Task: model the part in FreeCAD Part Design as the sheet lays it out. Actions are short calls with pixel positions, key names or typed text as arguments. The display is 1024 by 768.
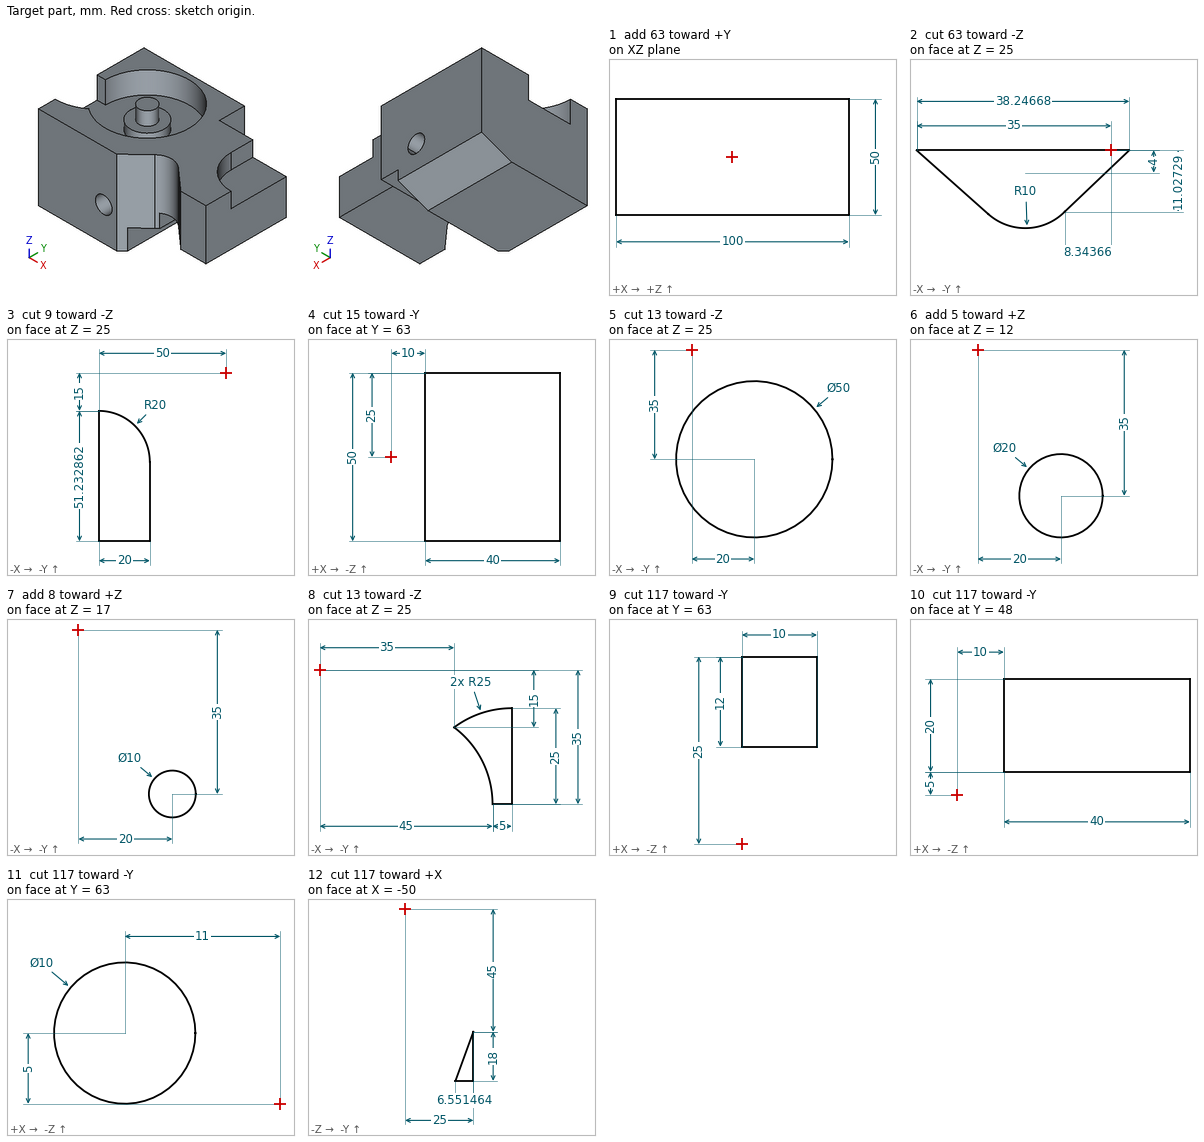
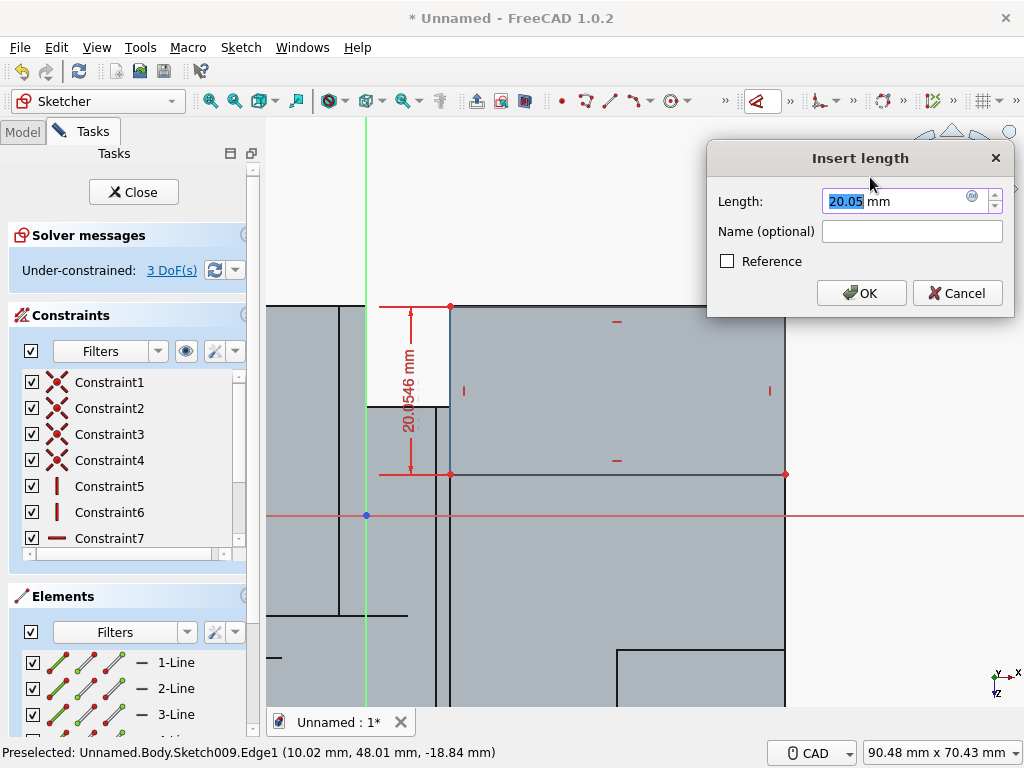
text(20)
key(Return)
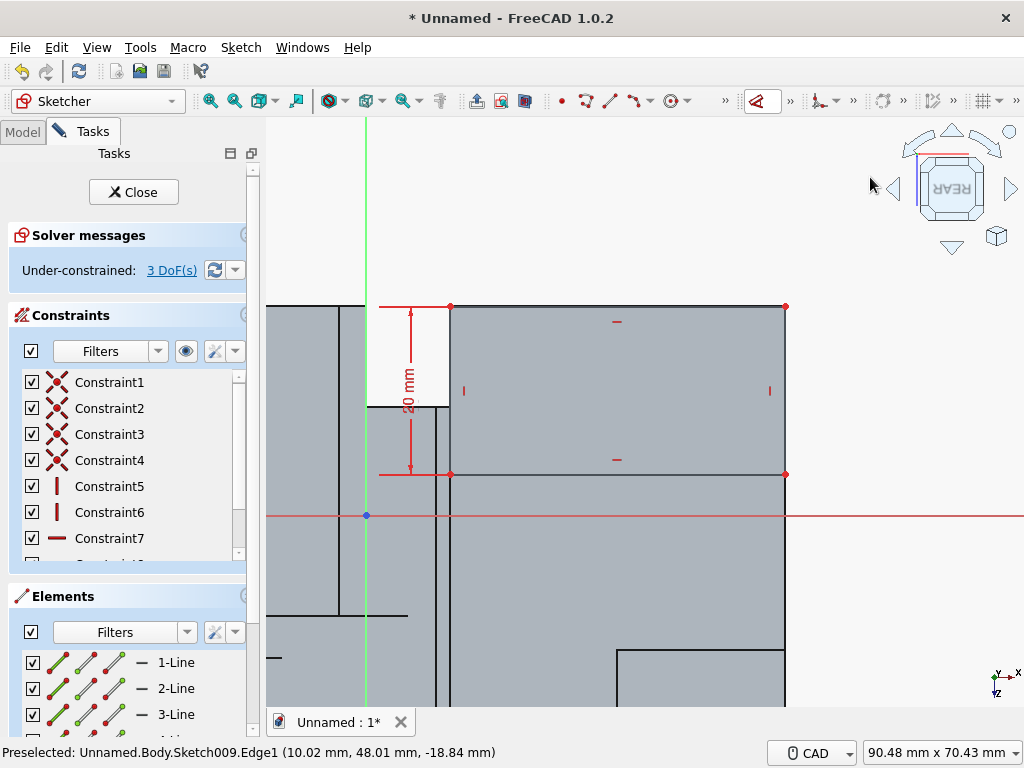
click(550, 475)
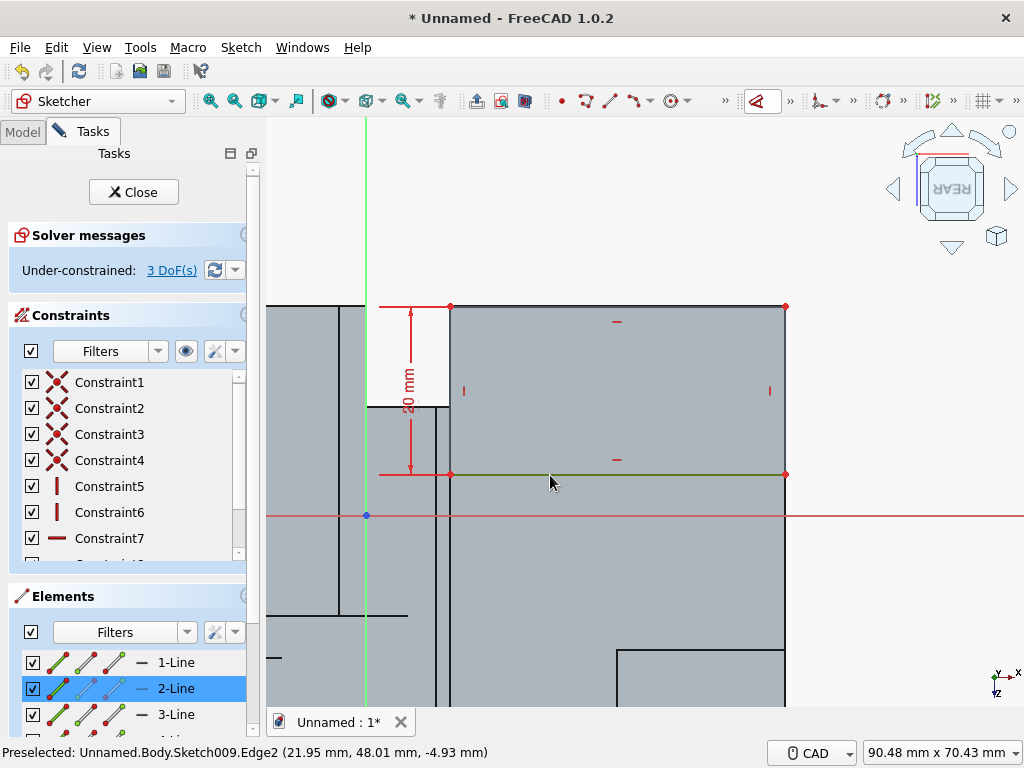
key(l)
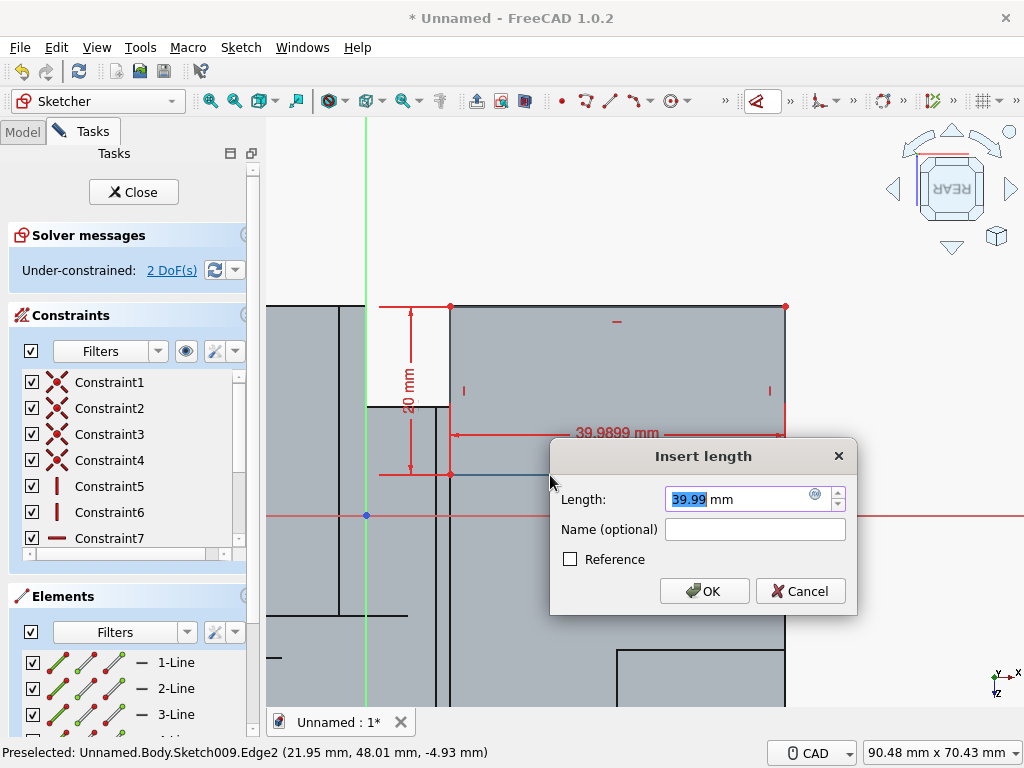
text(40)
key(Return)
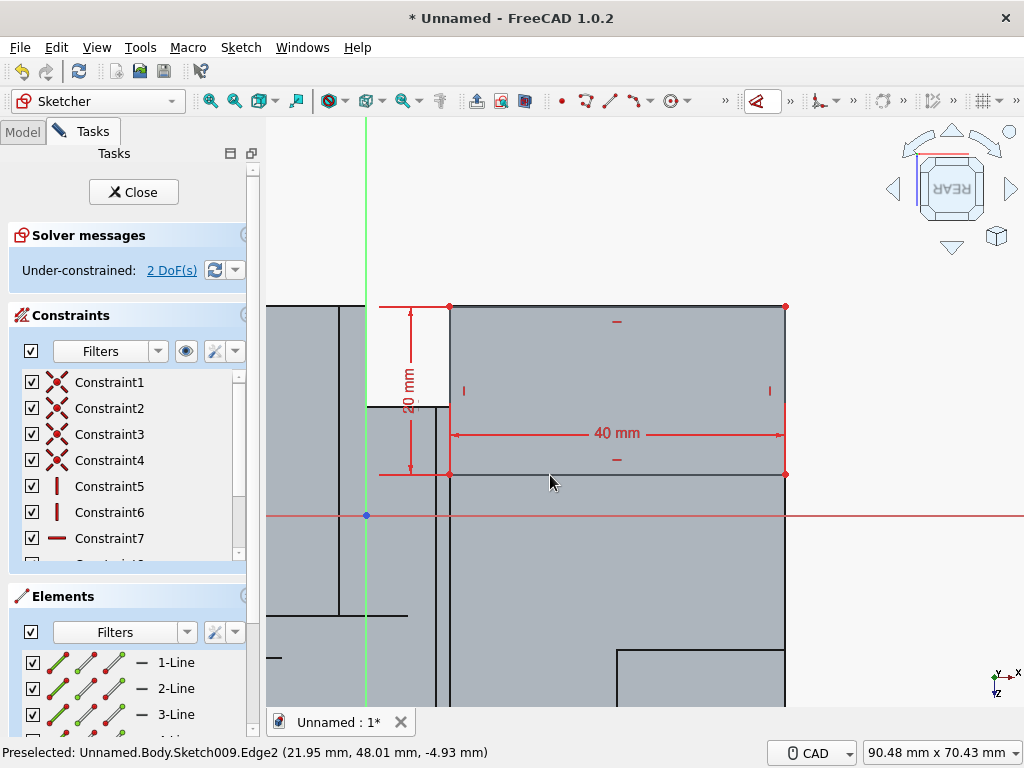
click(450, 475)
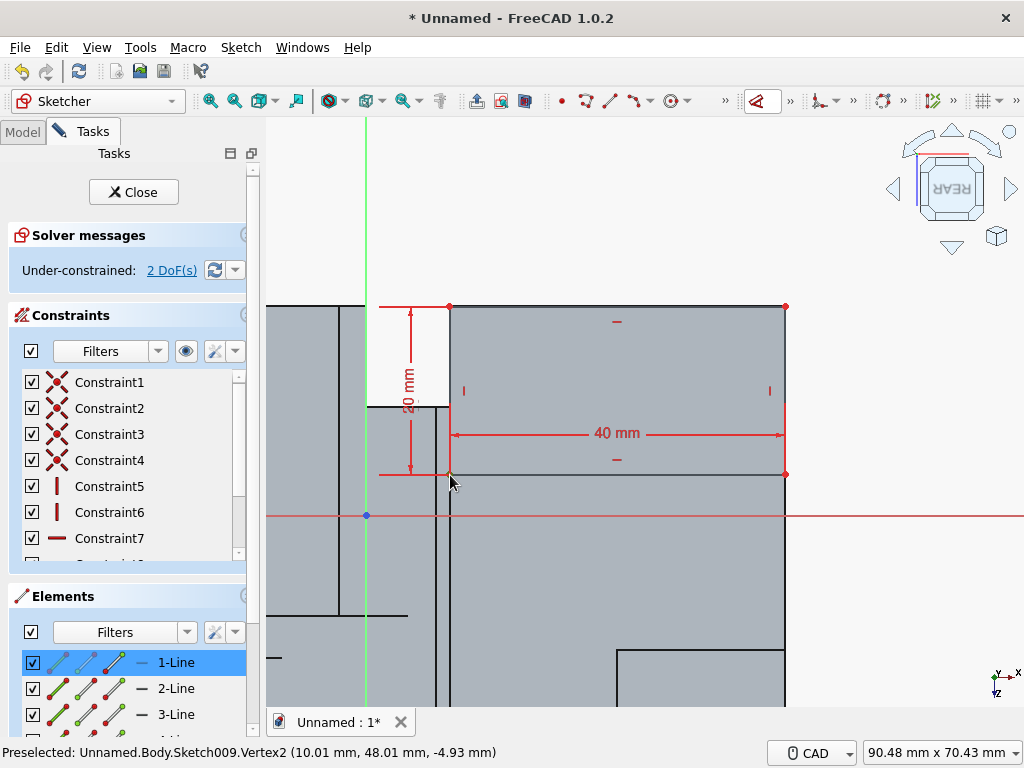
key(i)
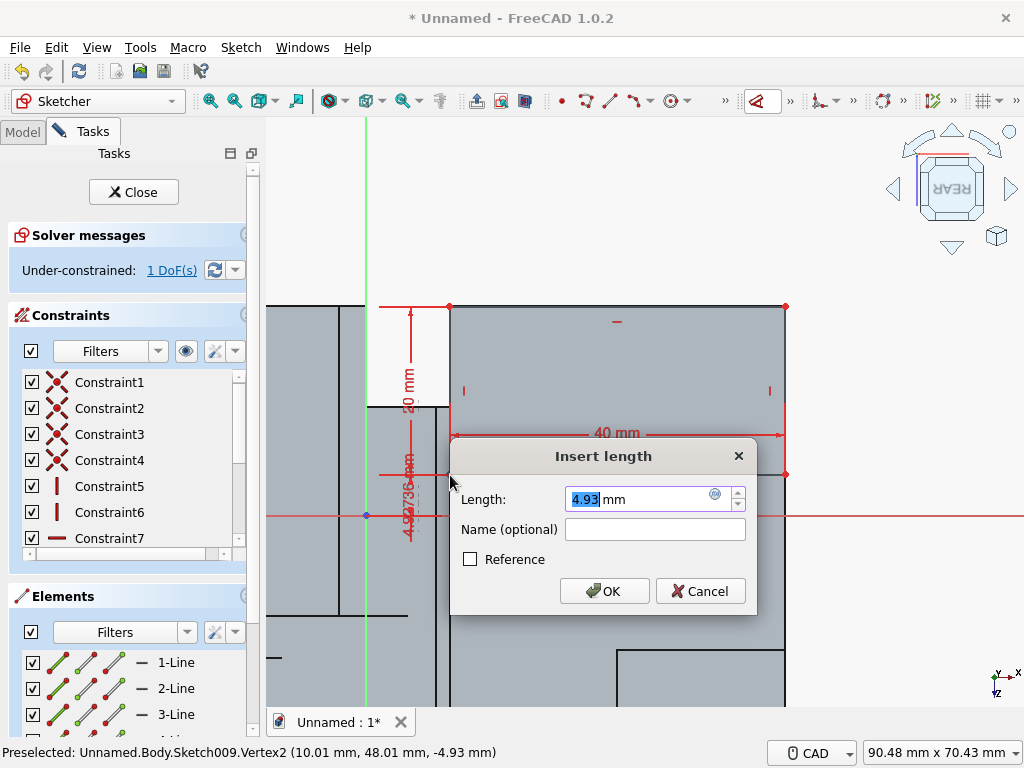
text(5)
key(Return)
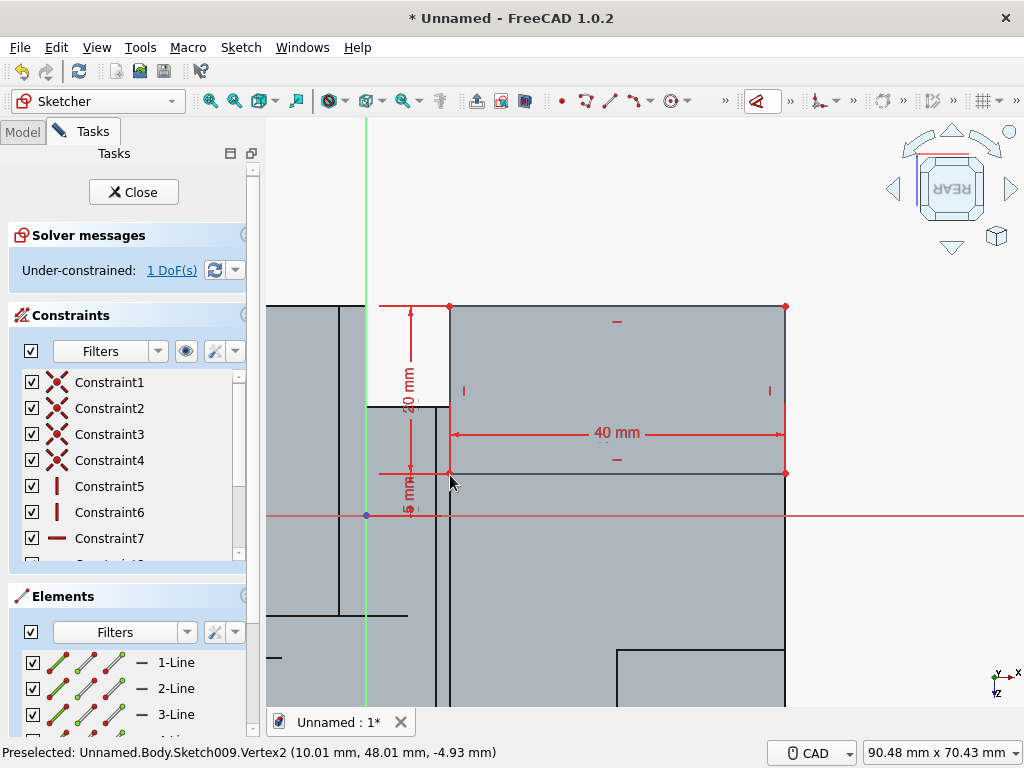
click(450, 306)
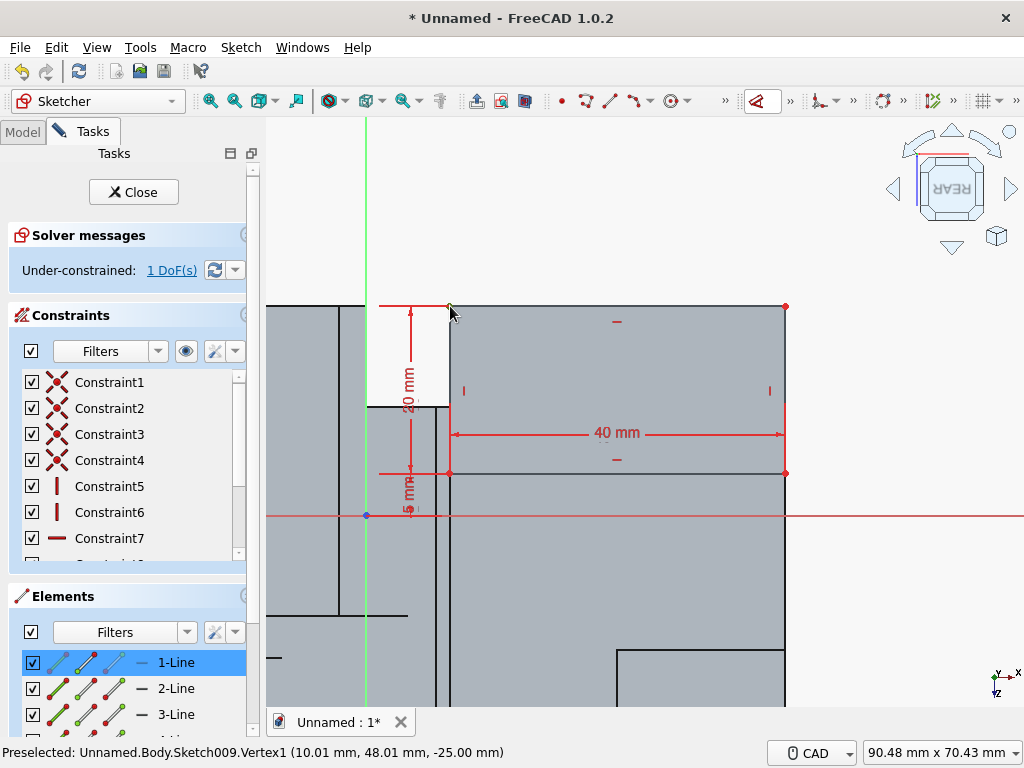
click(776, 102)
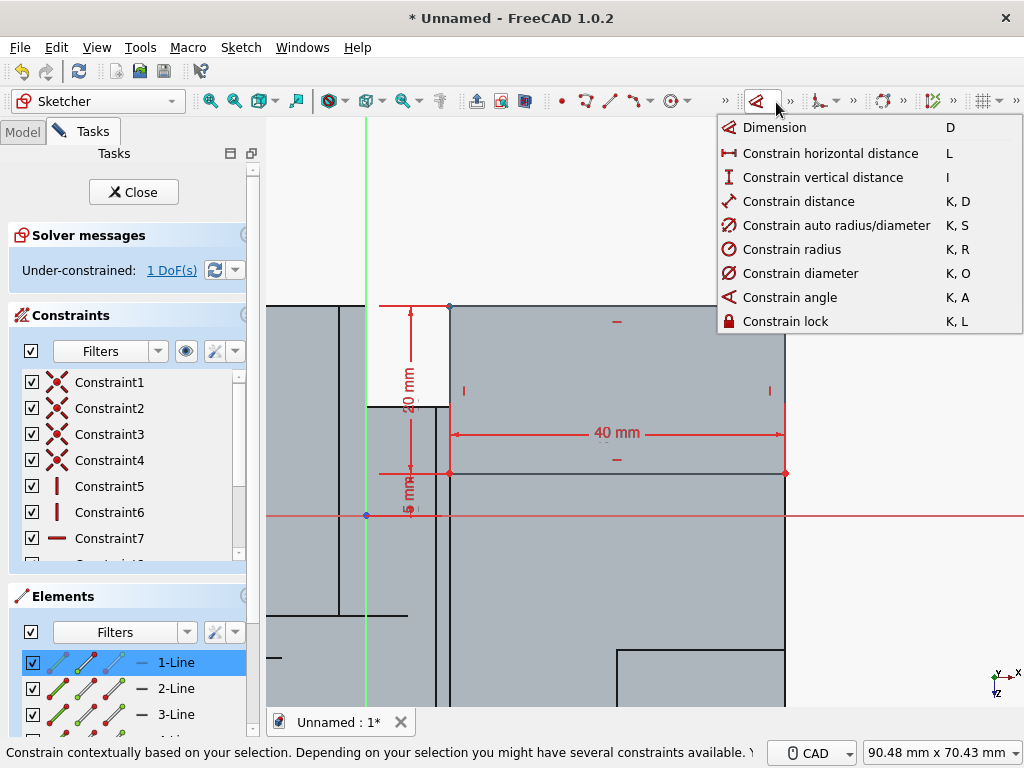
click(870, 153)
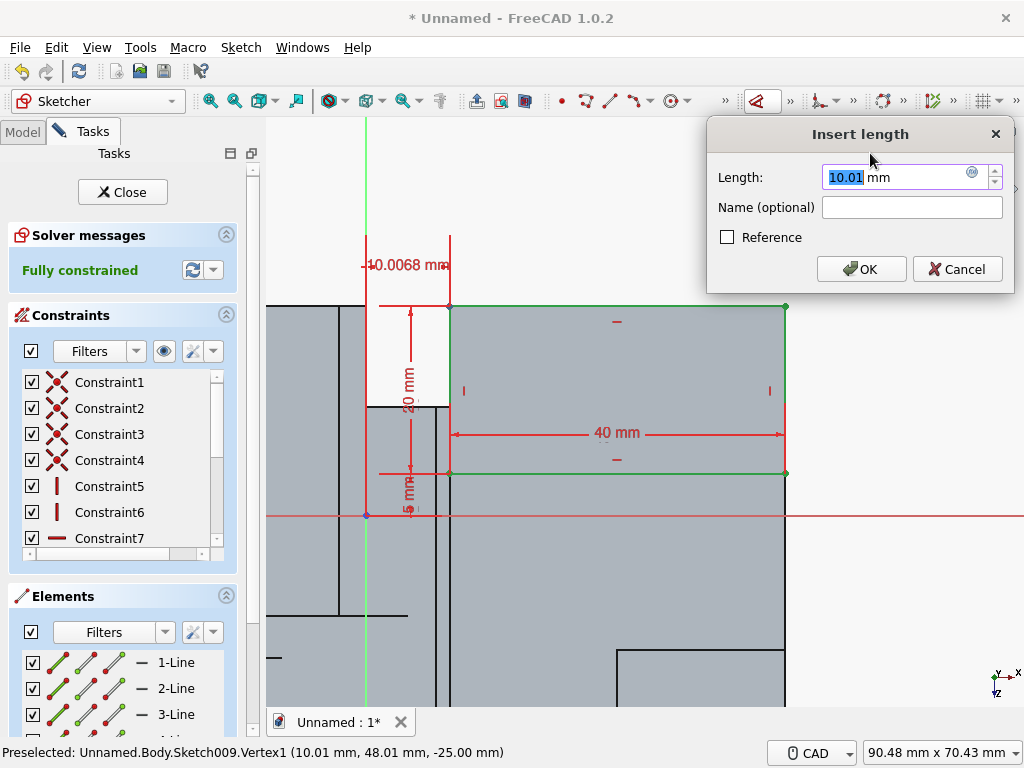
text(10)
key(Return)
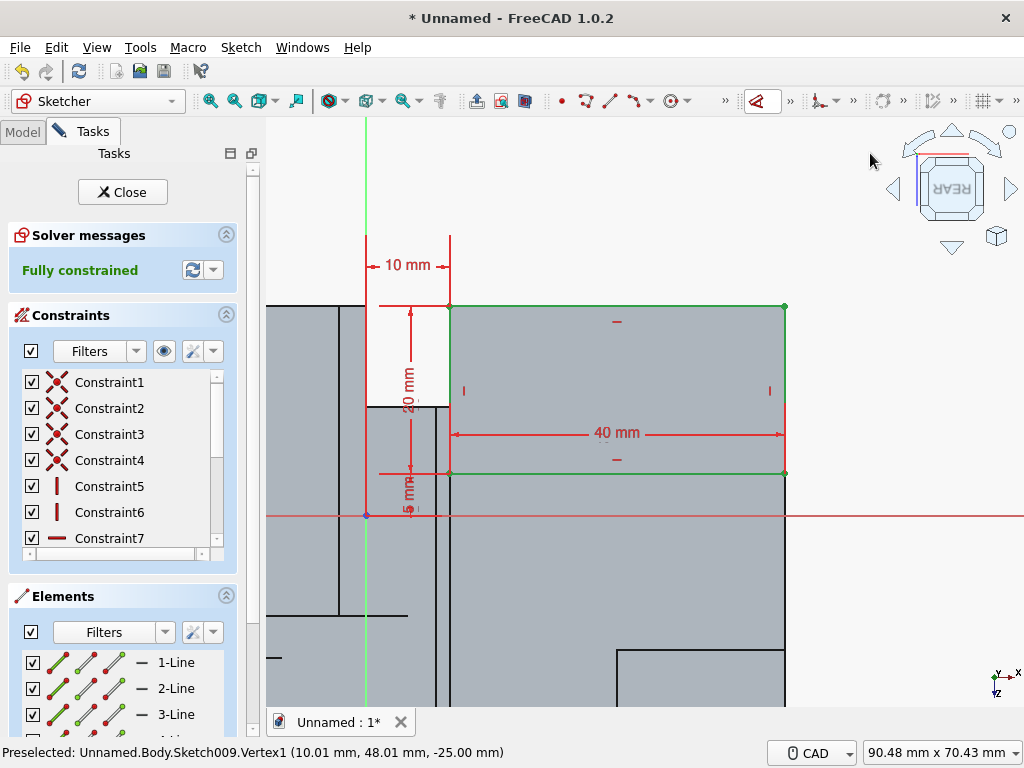
click(123, 192)